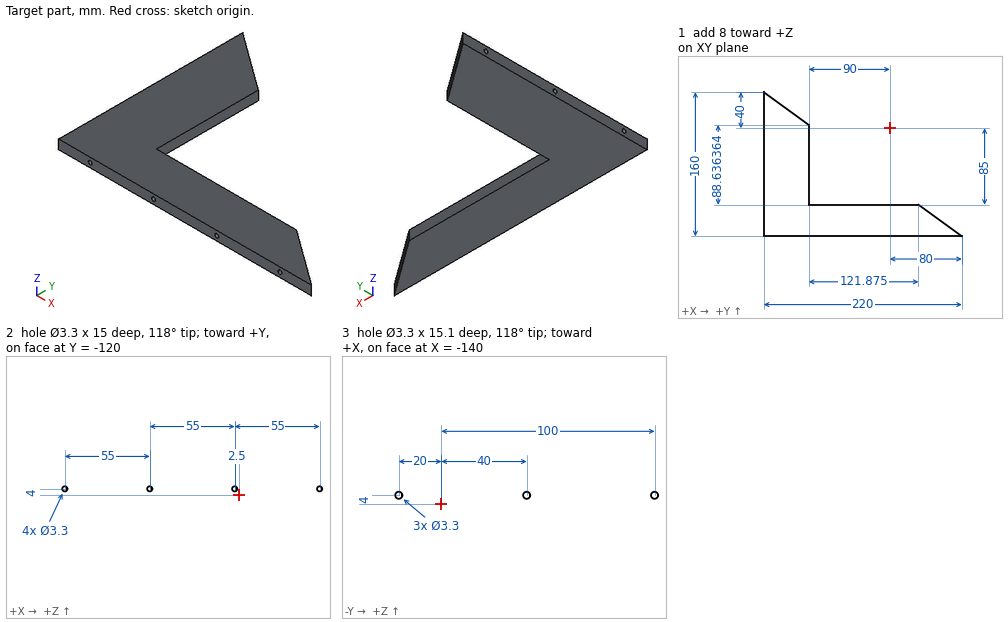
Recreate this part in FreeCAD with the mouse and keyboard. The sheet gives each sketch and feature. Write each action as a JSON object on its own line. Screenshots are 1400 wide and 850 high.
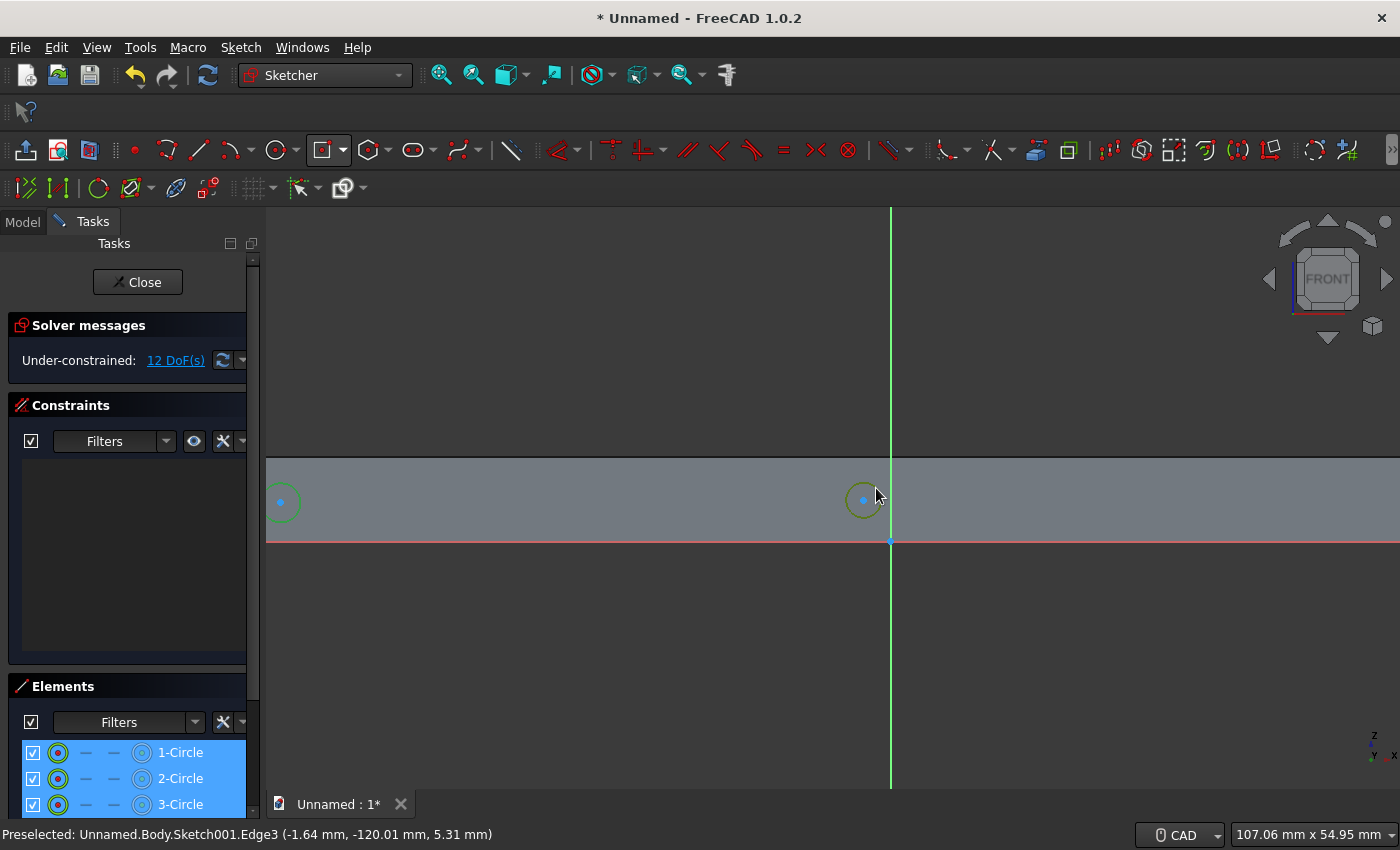
{"action": "scroll", "coordinate": [876, 490], "scroll_direction": "down", "scroll_amount": 5}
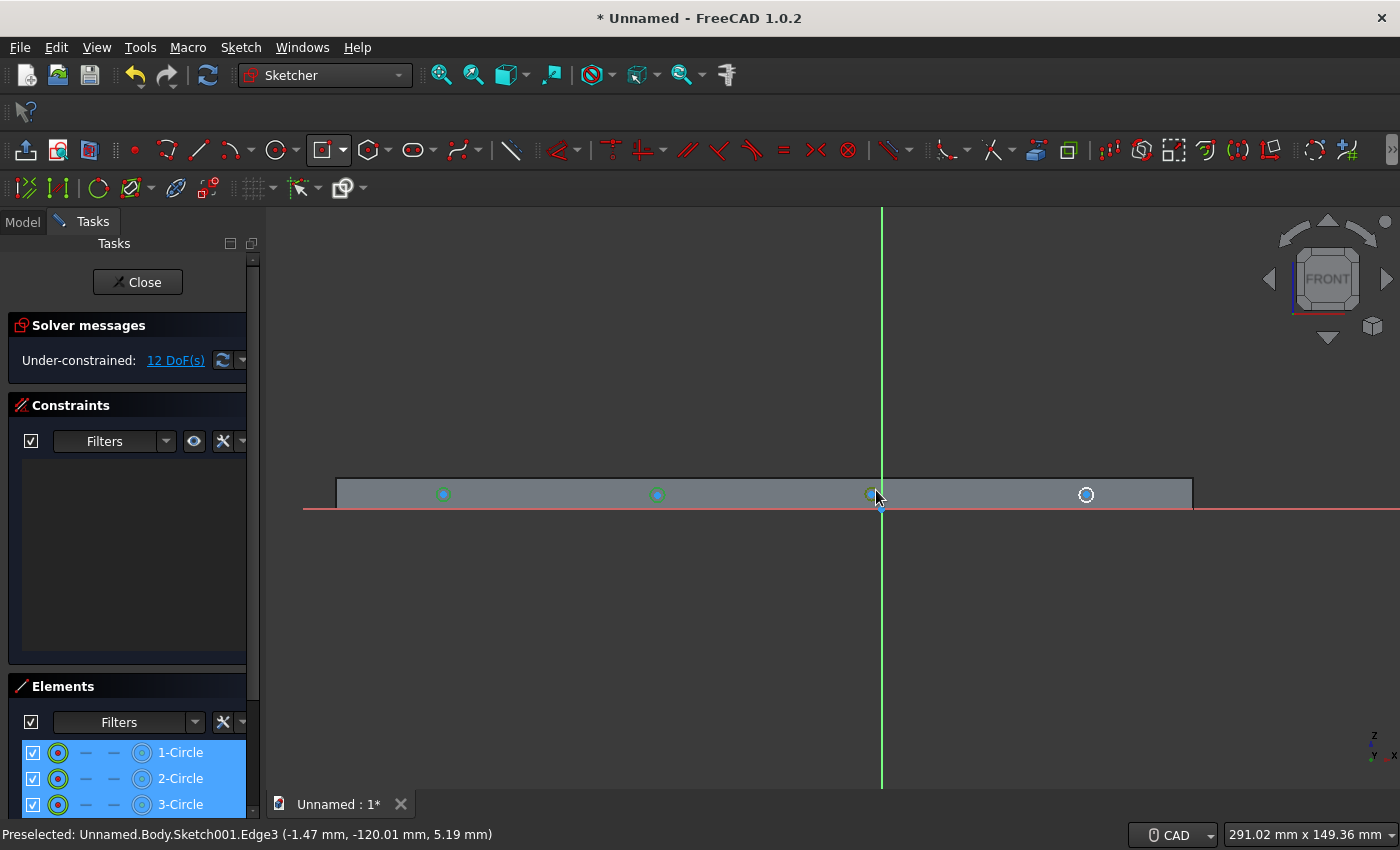
{"action": "scroll", "coordinate": [1091, 490], "scroll_direction": "up", "scroll_amount": 4}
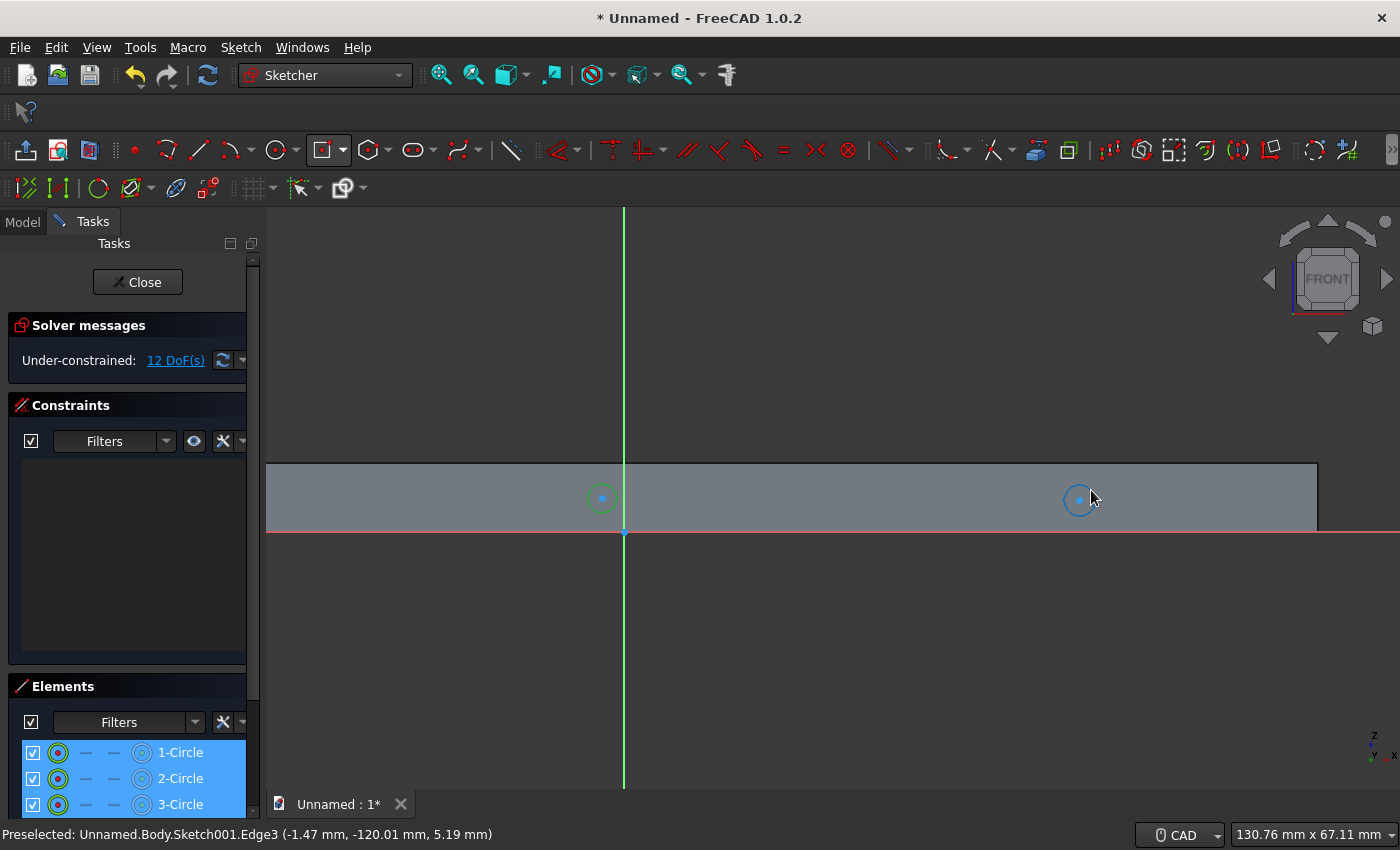
{"action": "left_click", "coordinate": [1091, 490]}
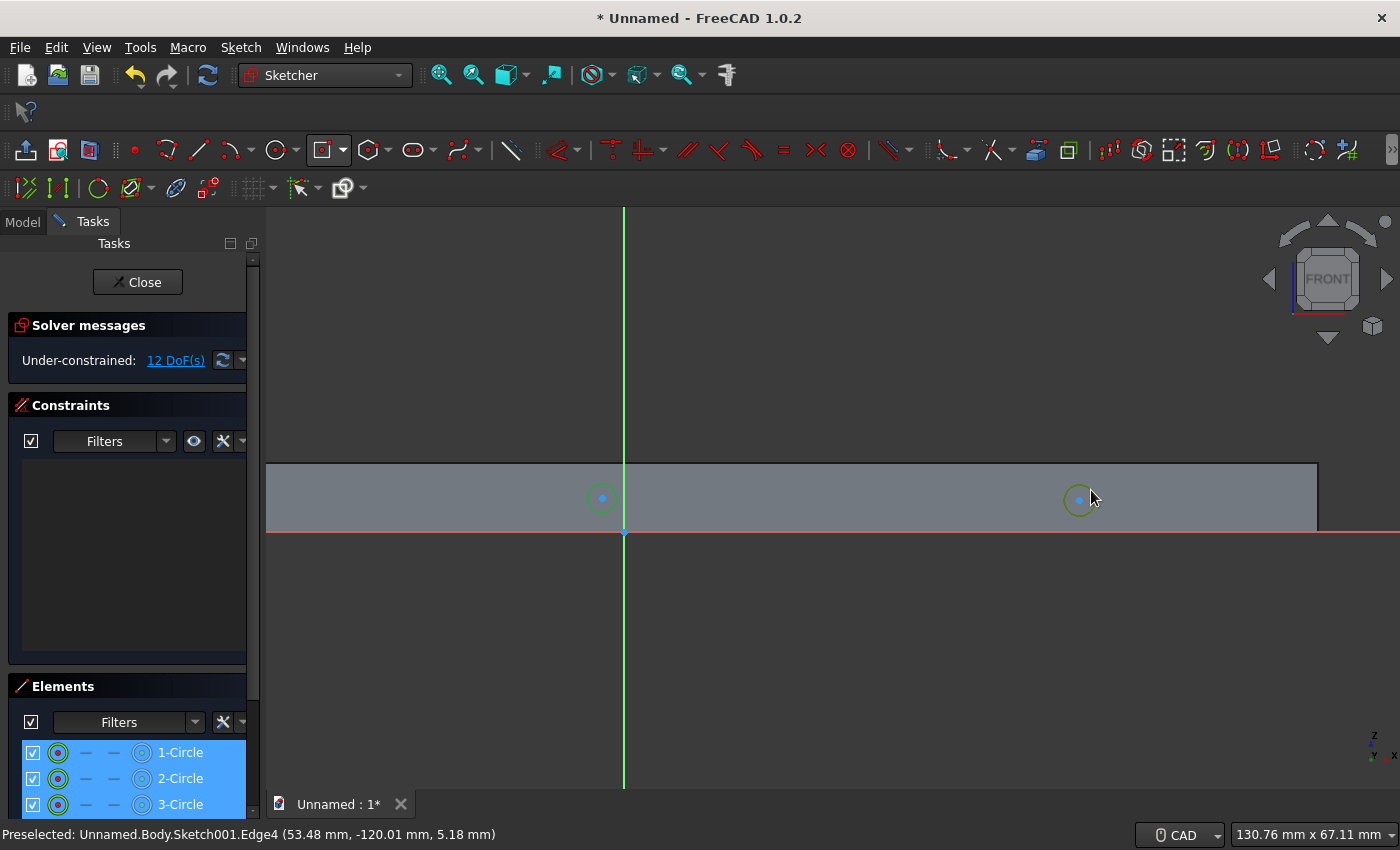
{"action": "key", "text": "e"}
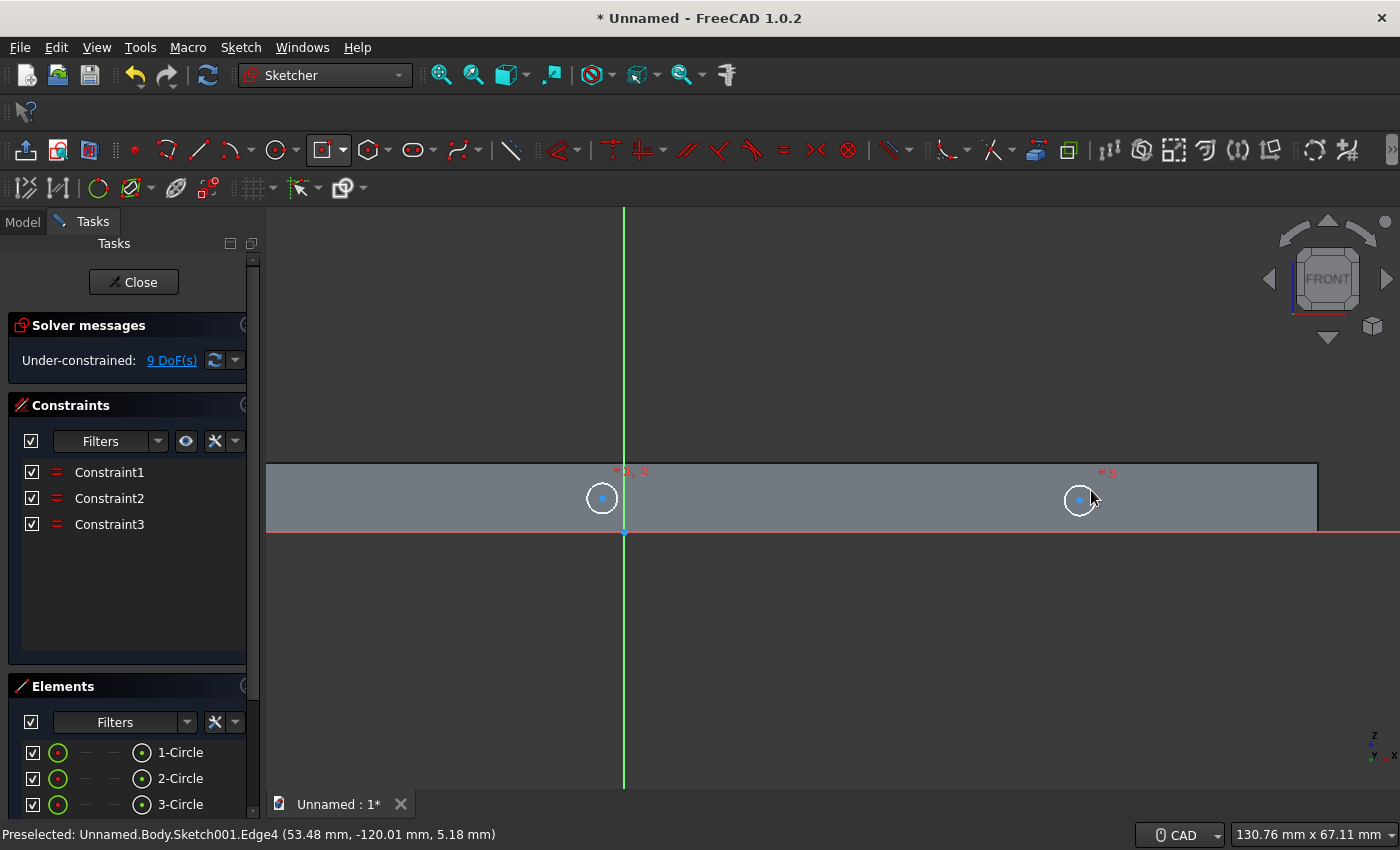
{"action": "scroll", "coordinate": [1091, 490], "scroll_direction": "down", "scroll_amount": 4}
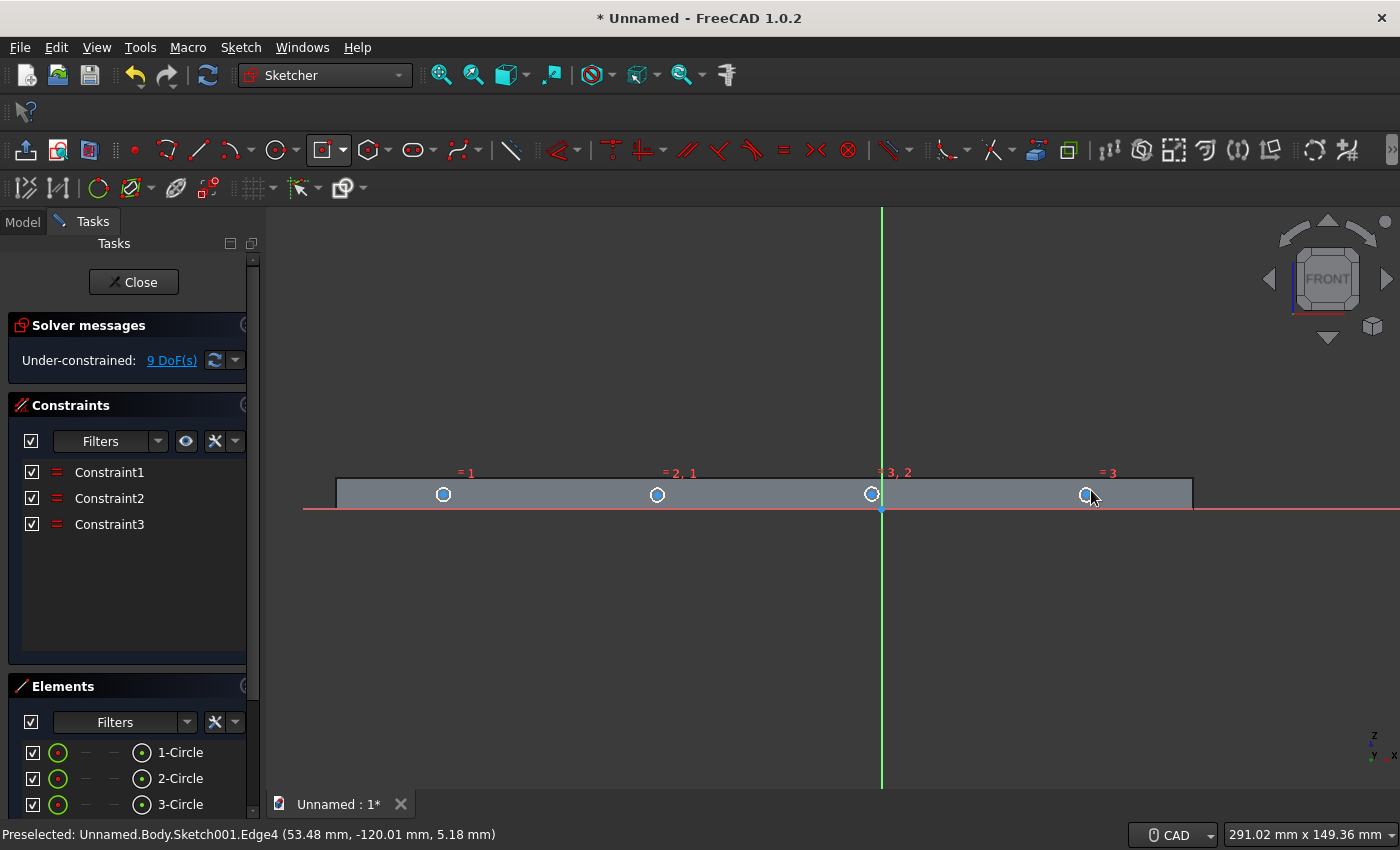
{"action": "left_click", "coordinate": [443, 495]}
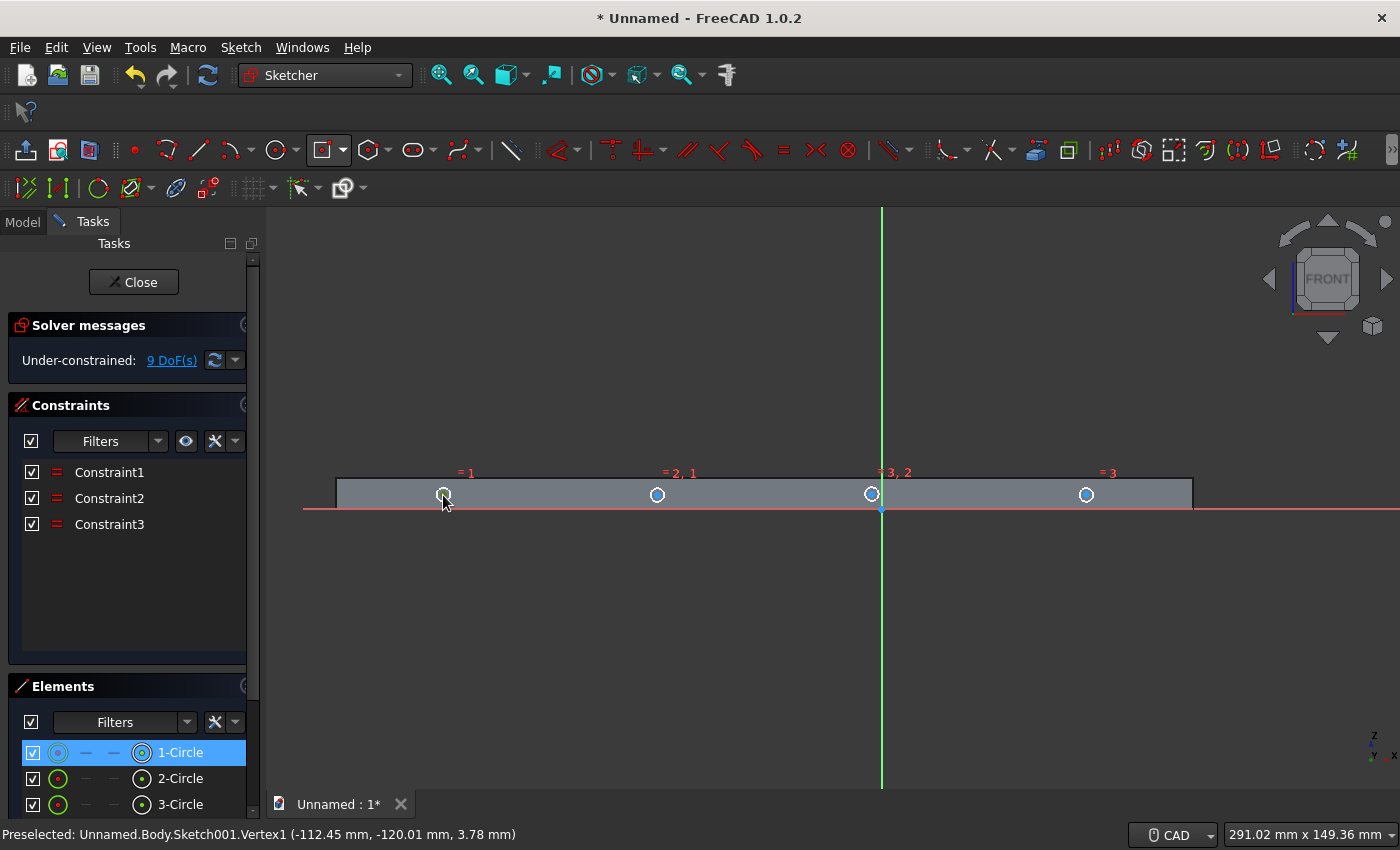
{"action": "left_click", "coordinate": [657, 495]}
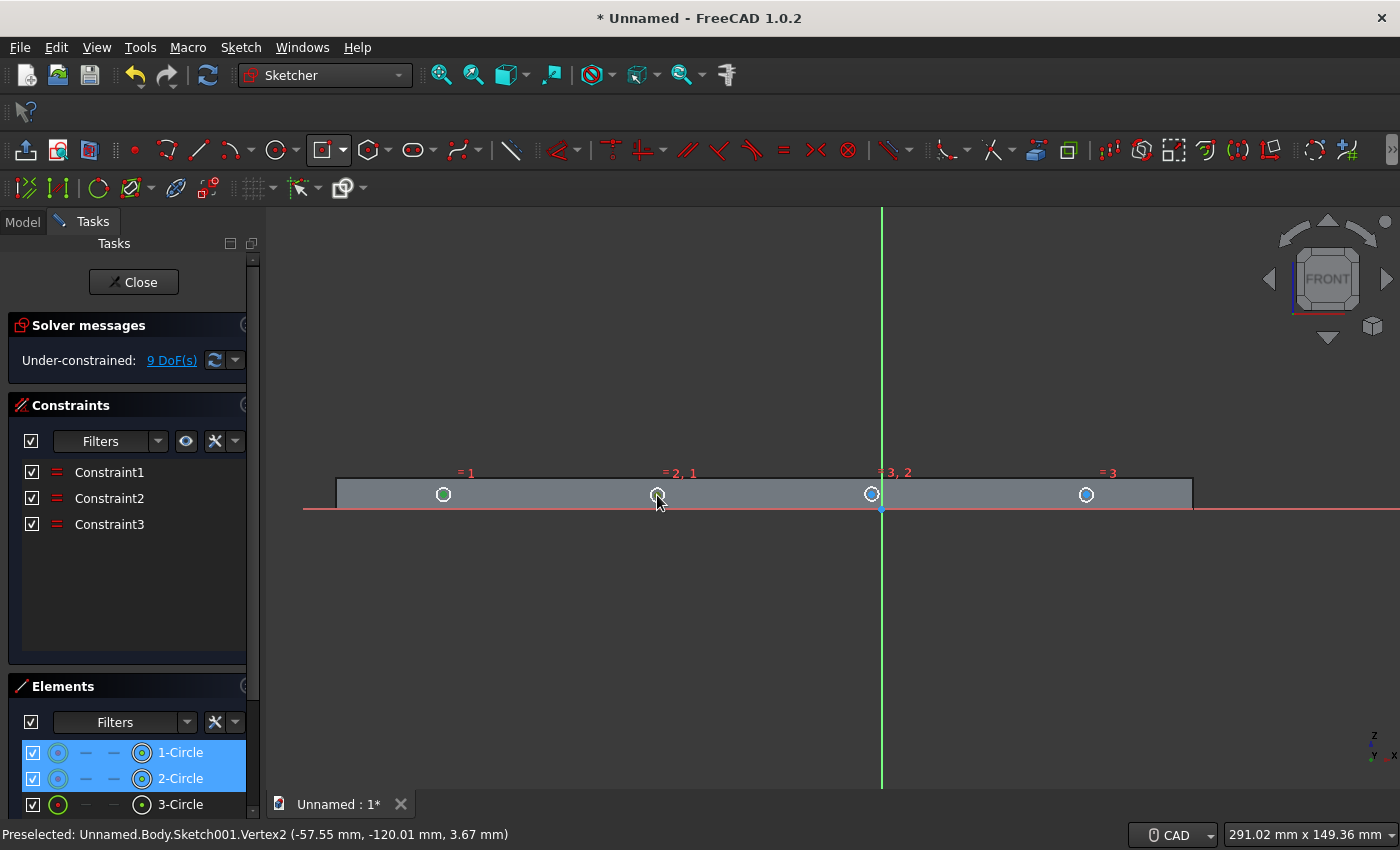
{"action": "key", "text": "h"}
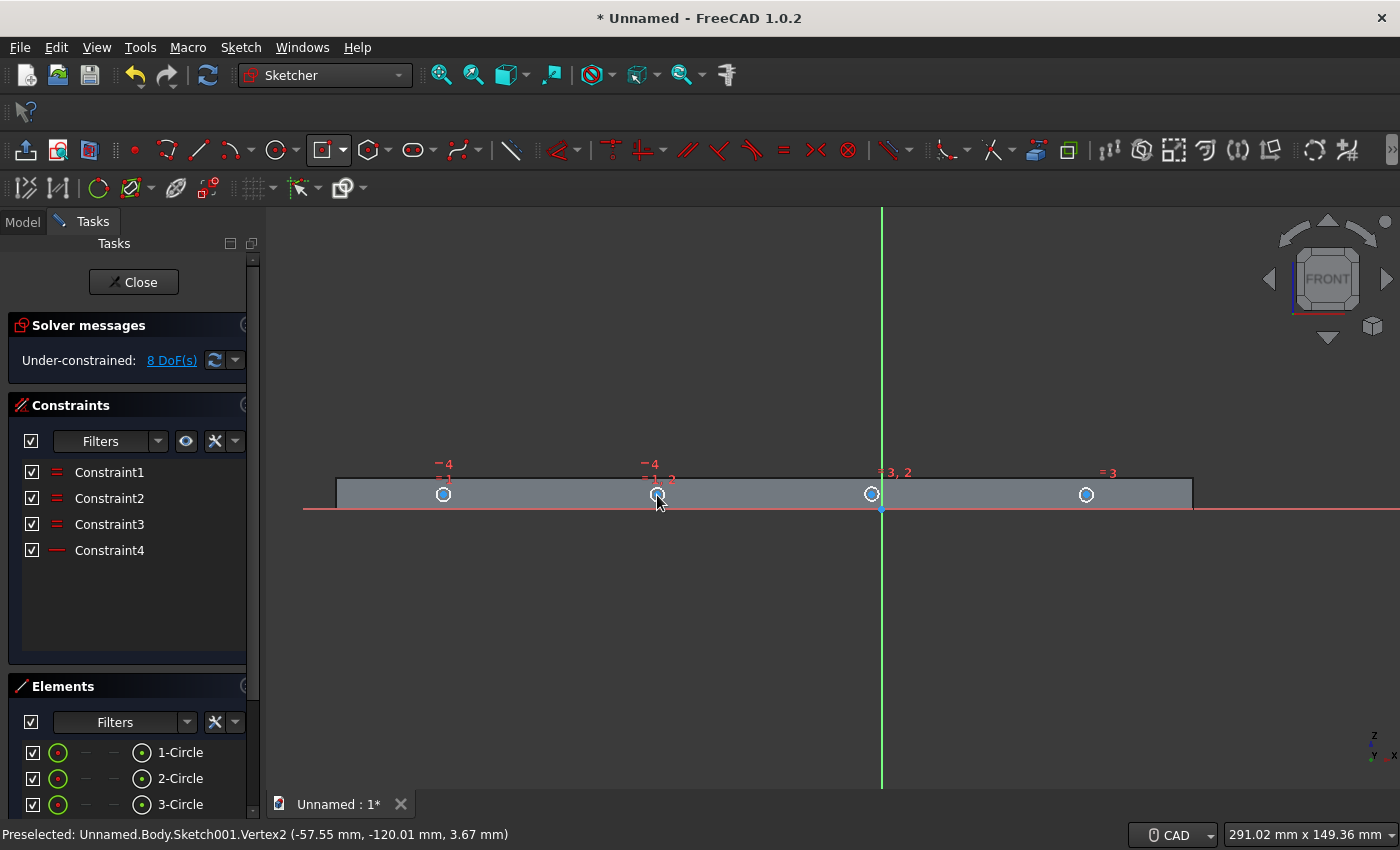
{"action": "left_click", "coordinate": [657, 495]}